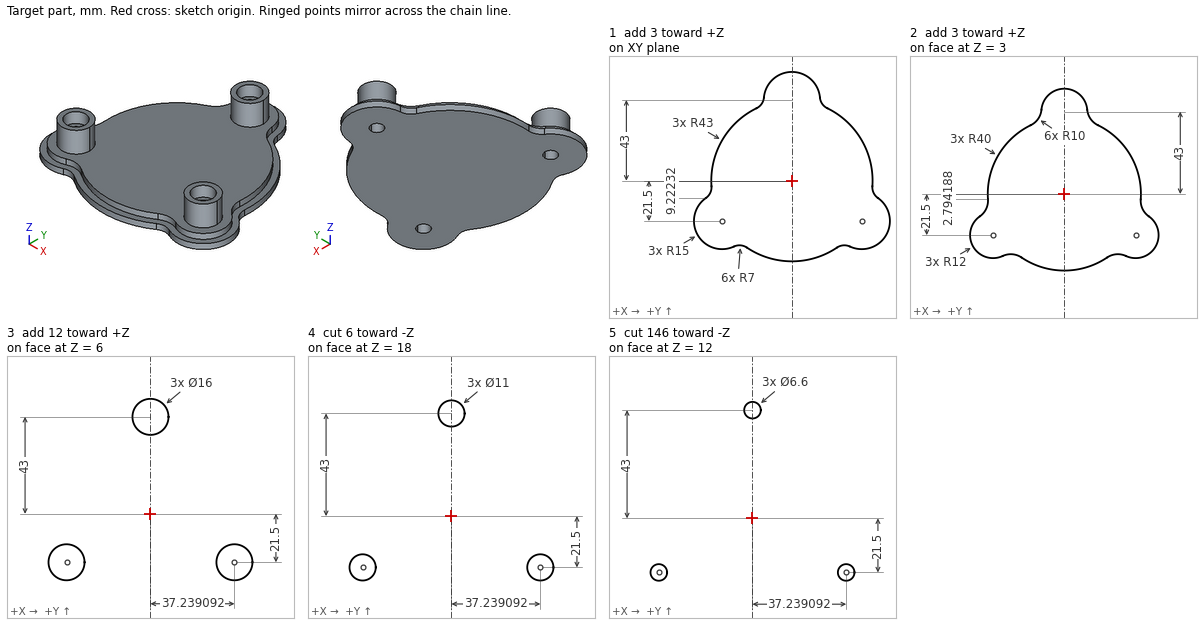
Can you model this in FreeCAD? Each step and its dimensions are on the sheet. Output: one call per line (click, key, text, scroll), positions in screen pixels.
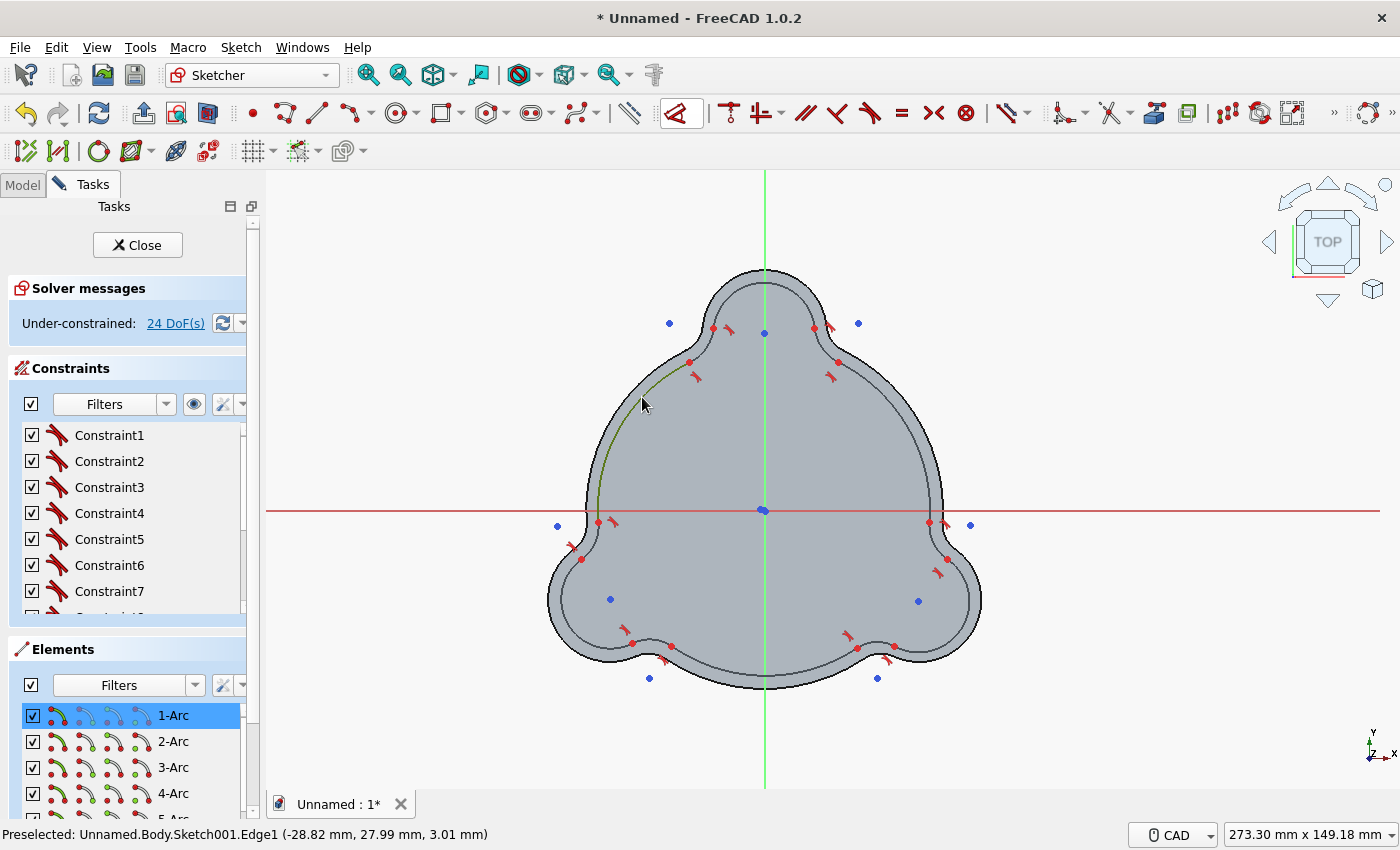
click(725, 671)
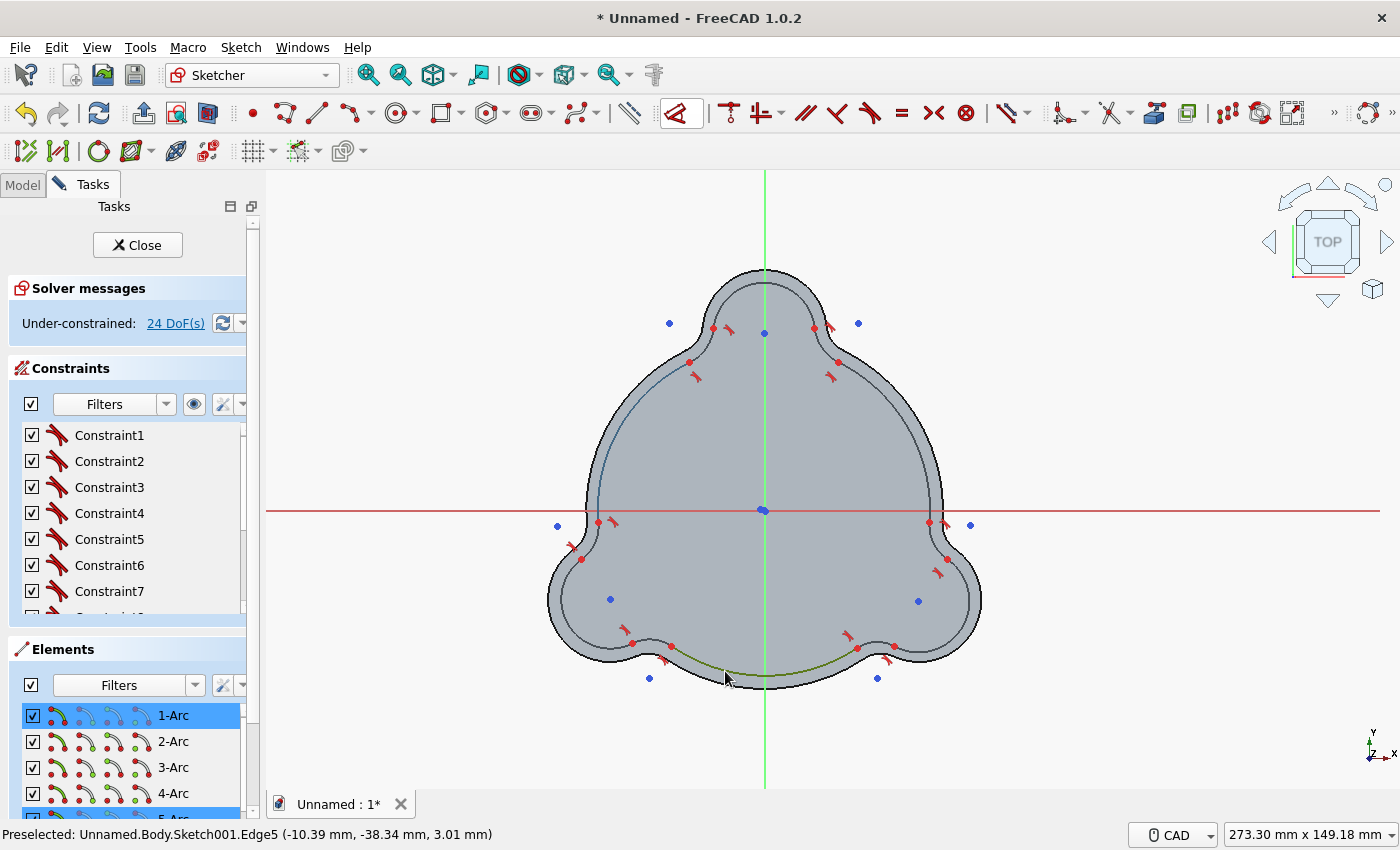
click(730, 114)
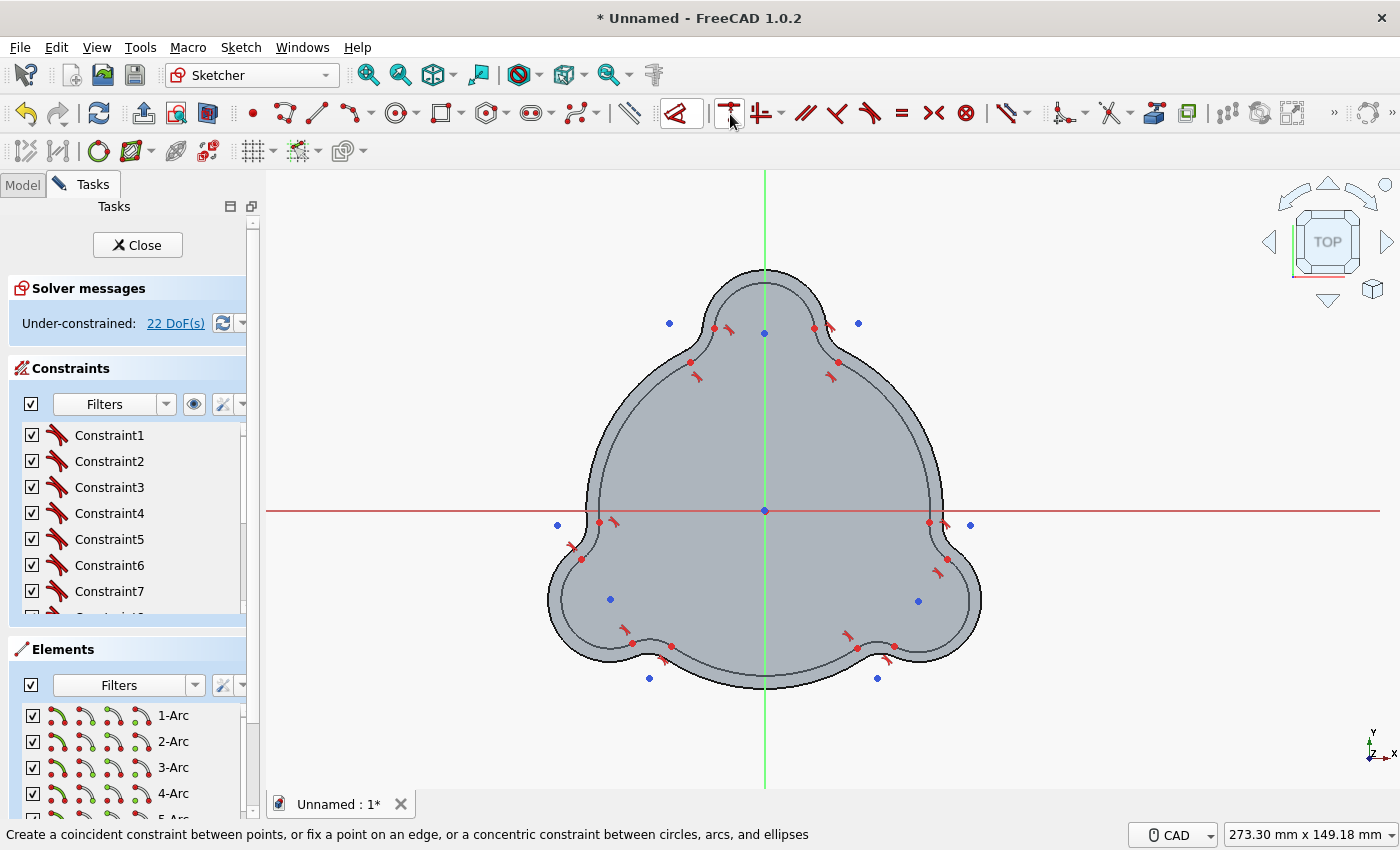
click(644, 398)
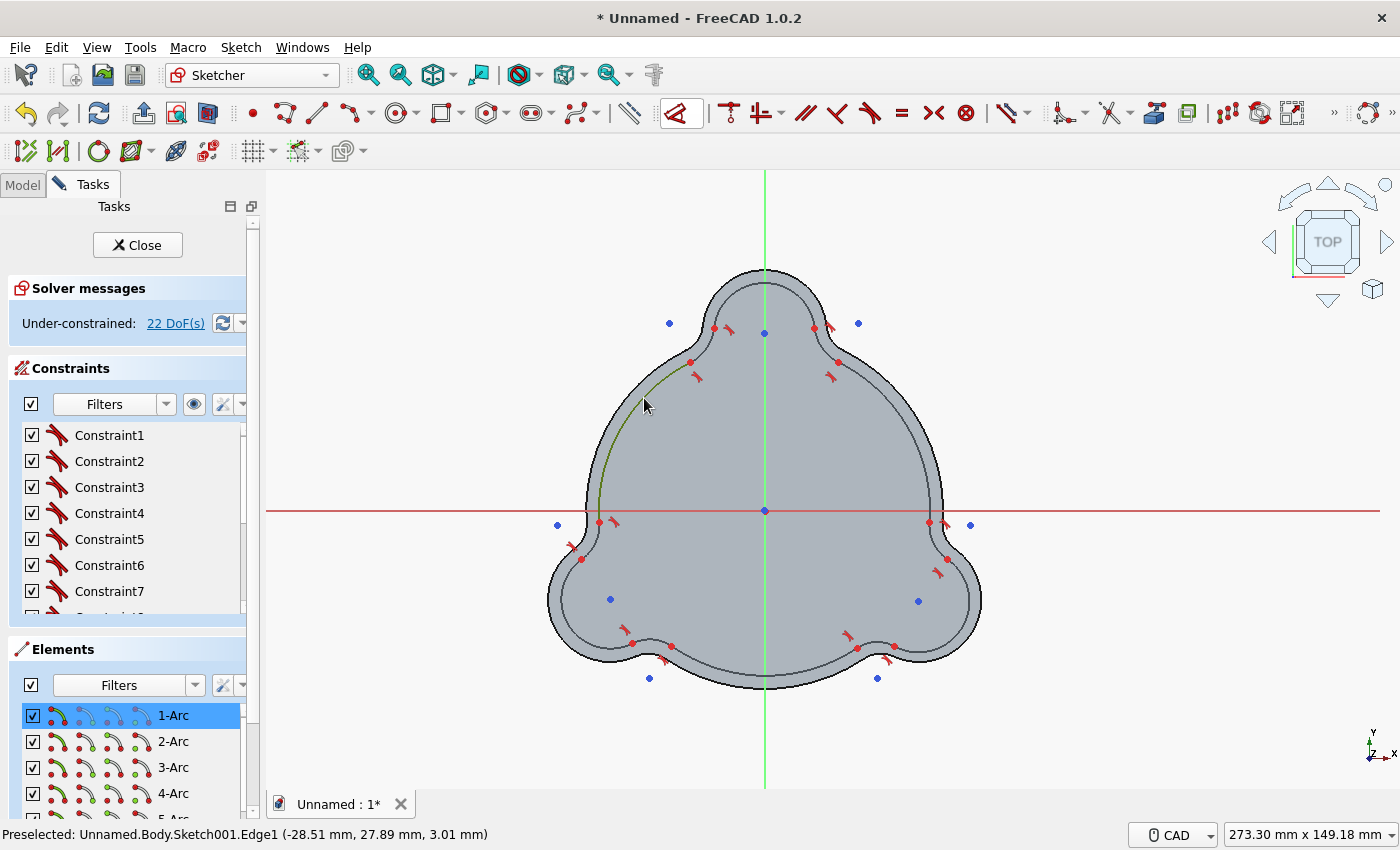
click(924, 465)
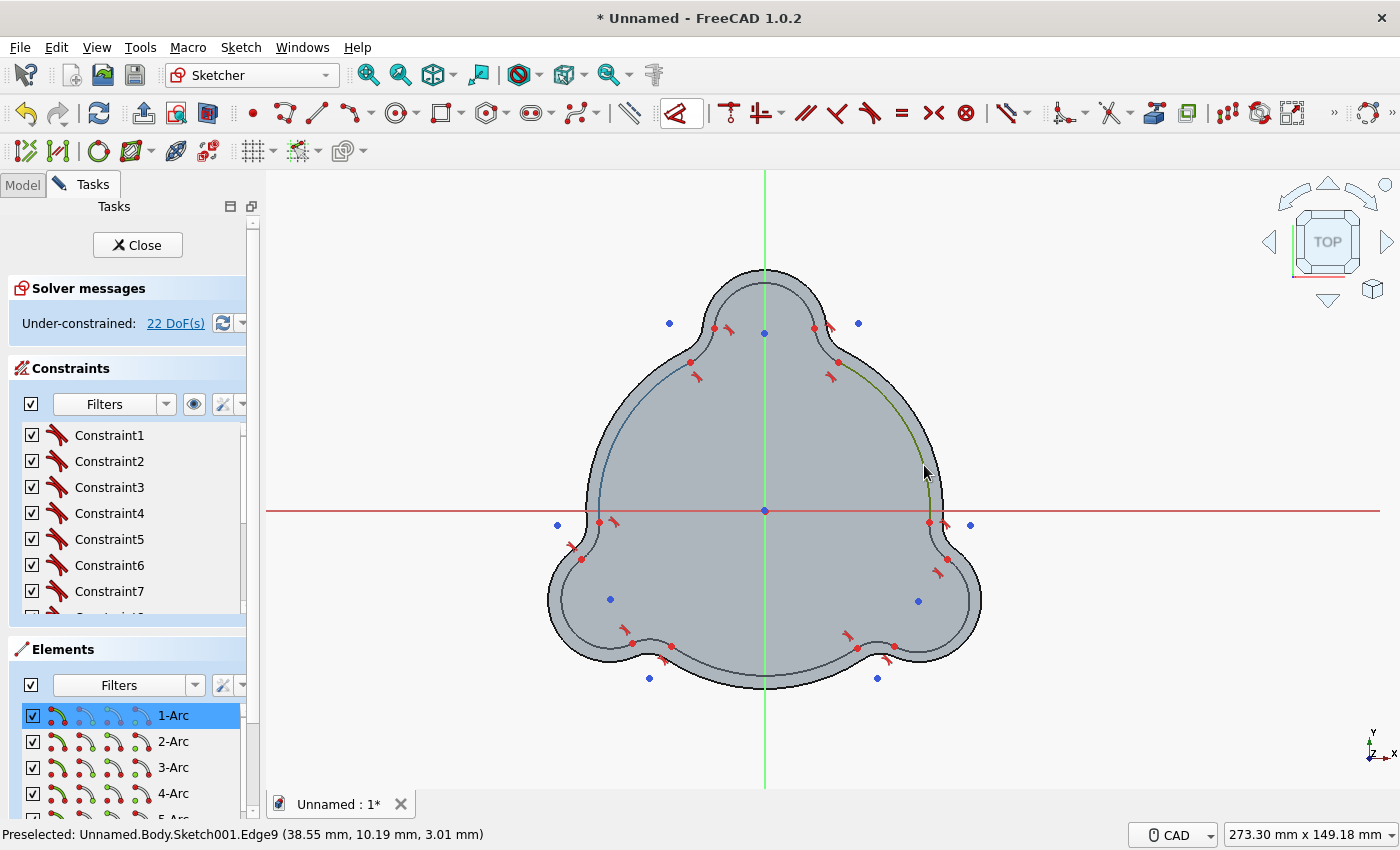
click(730, 114)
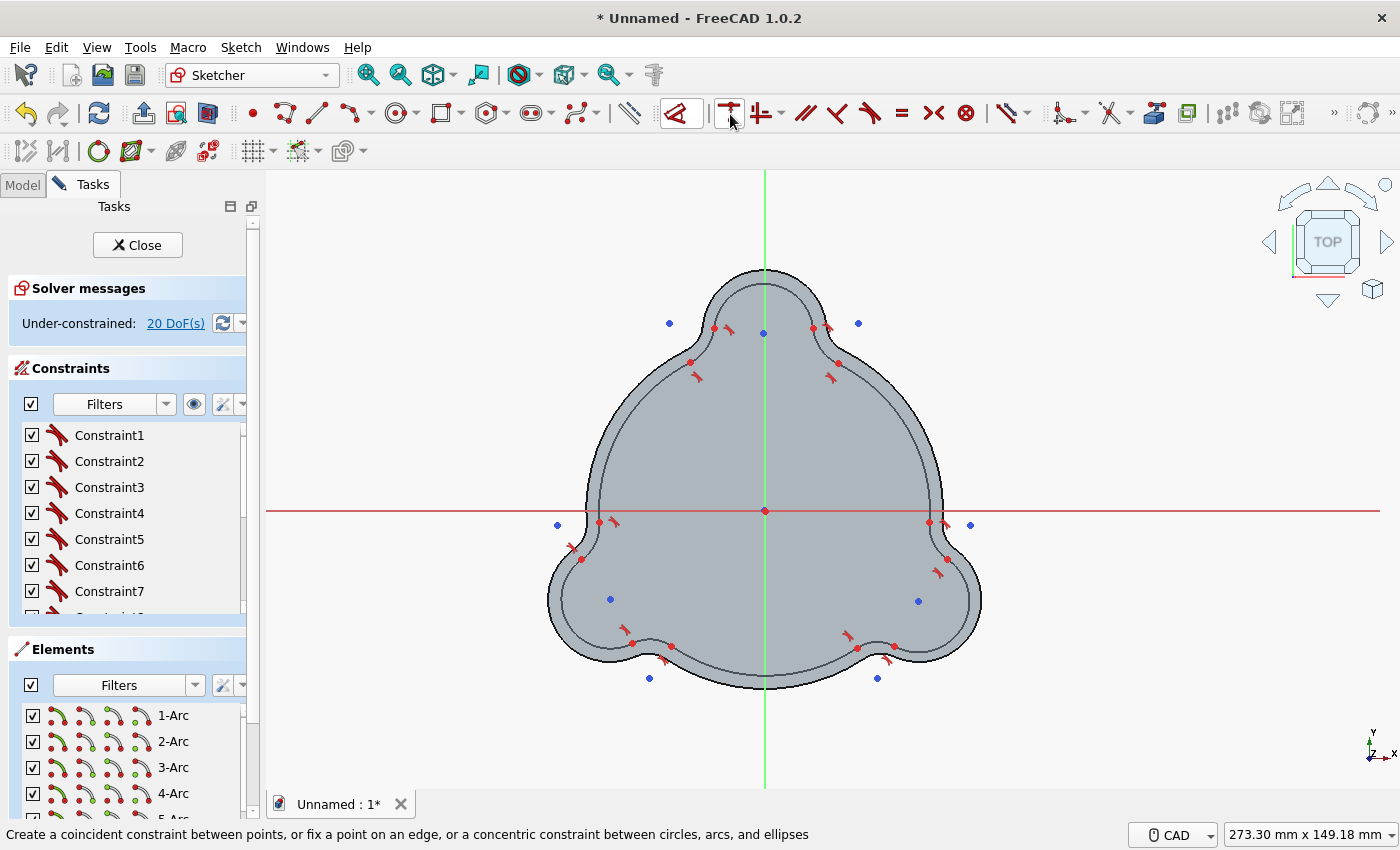
drag(755, 501, 776, 521)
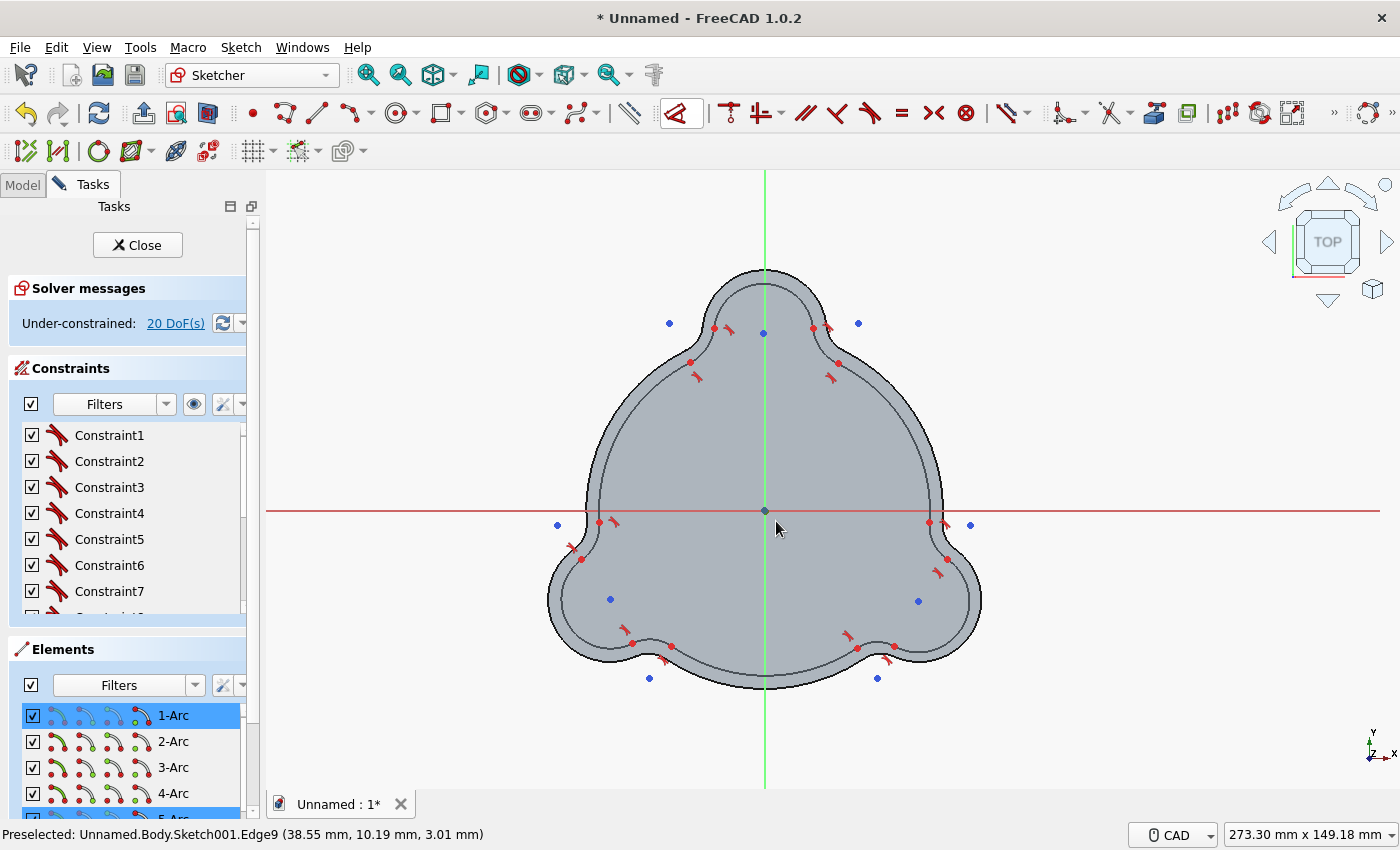
key(c)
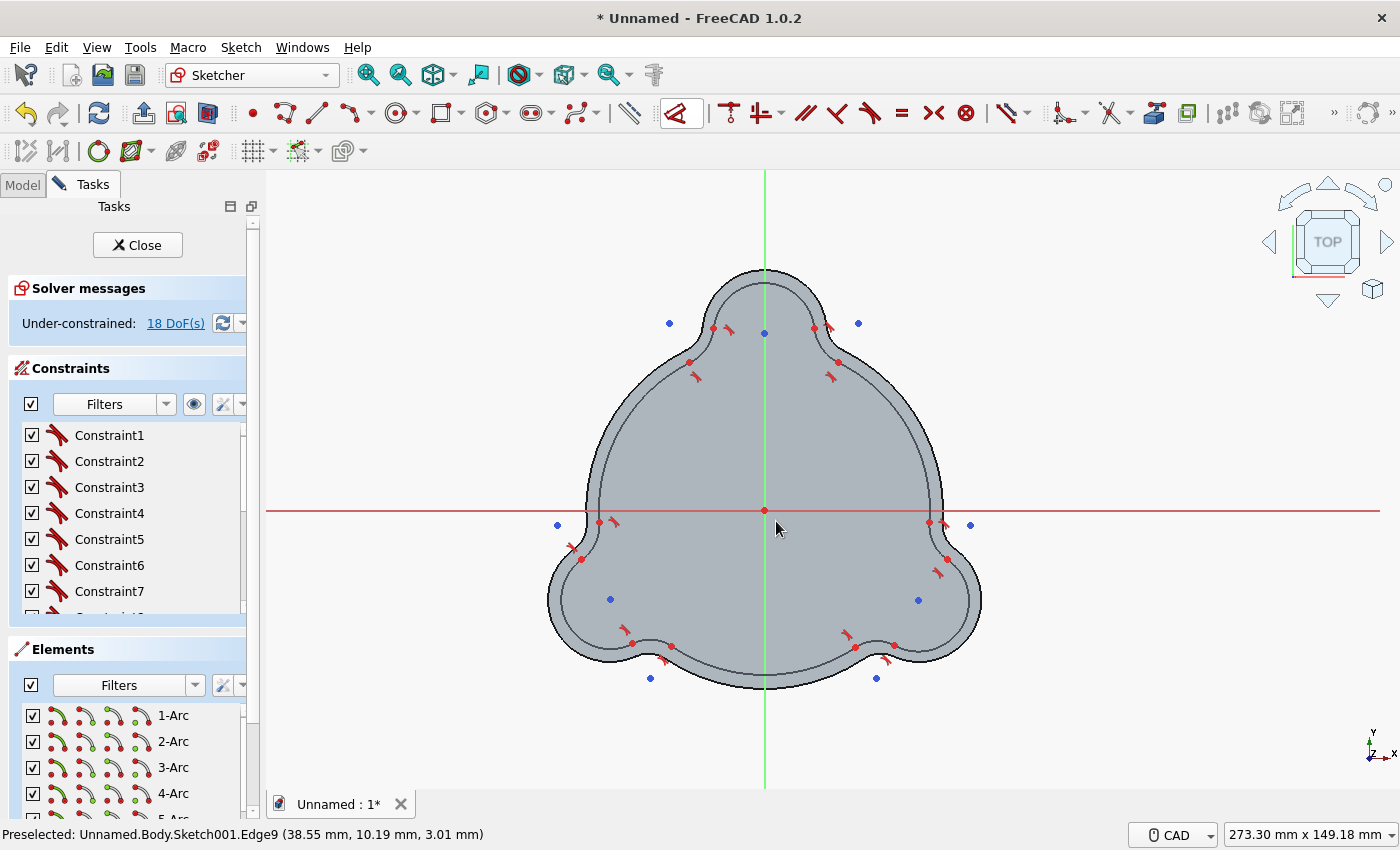
click(591, 551)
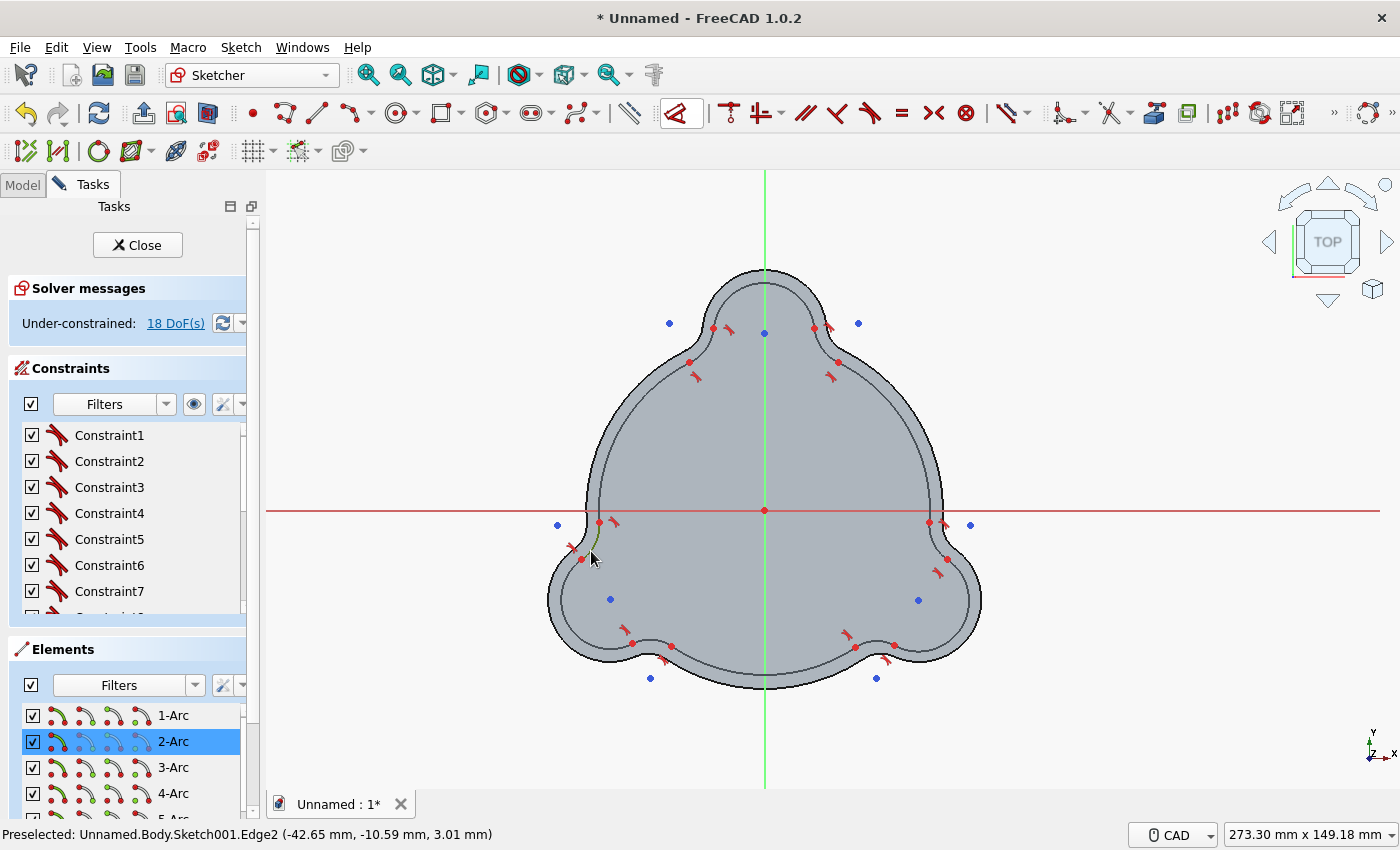
click(661, 641)